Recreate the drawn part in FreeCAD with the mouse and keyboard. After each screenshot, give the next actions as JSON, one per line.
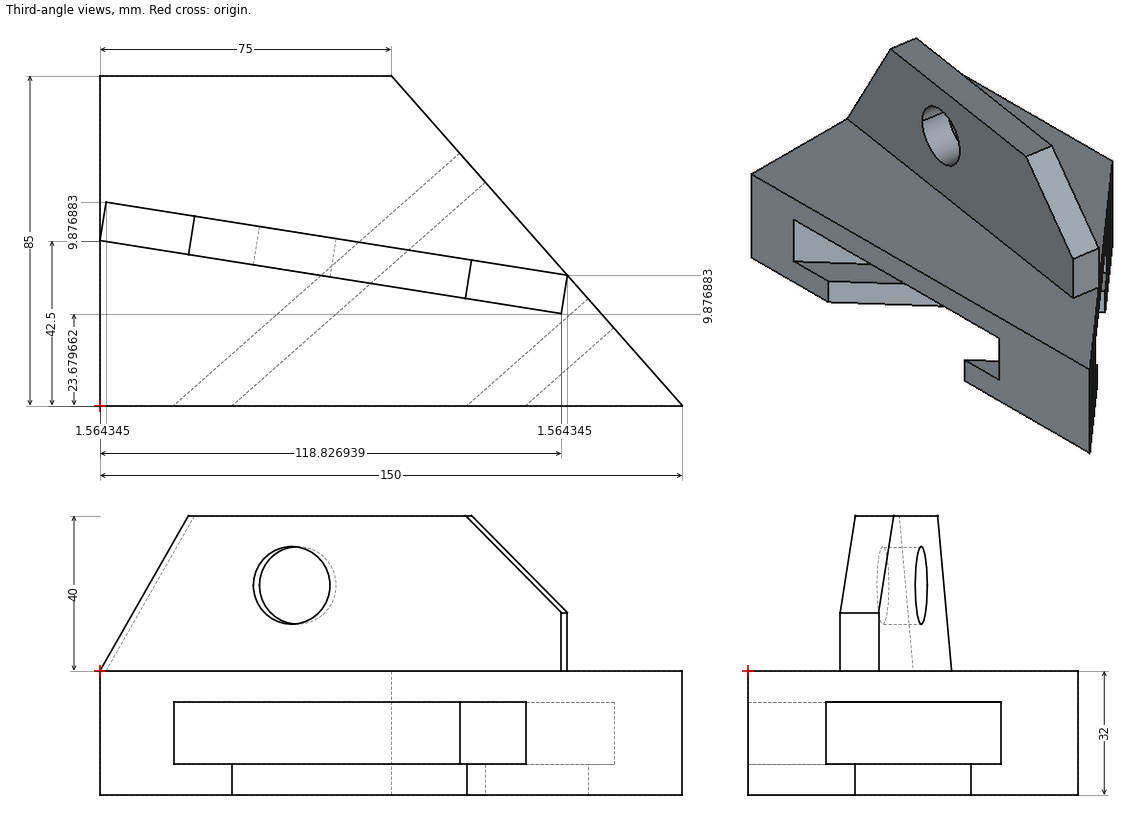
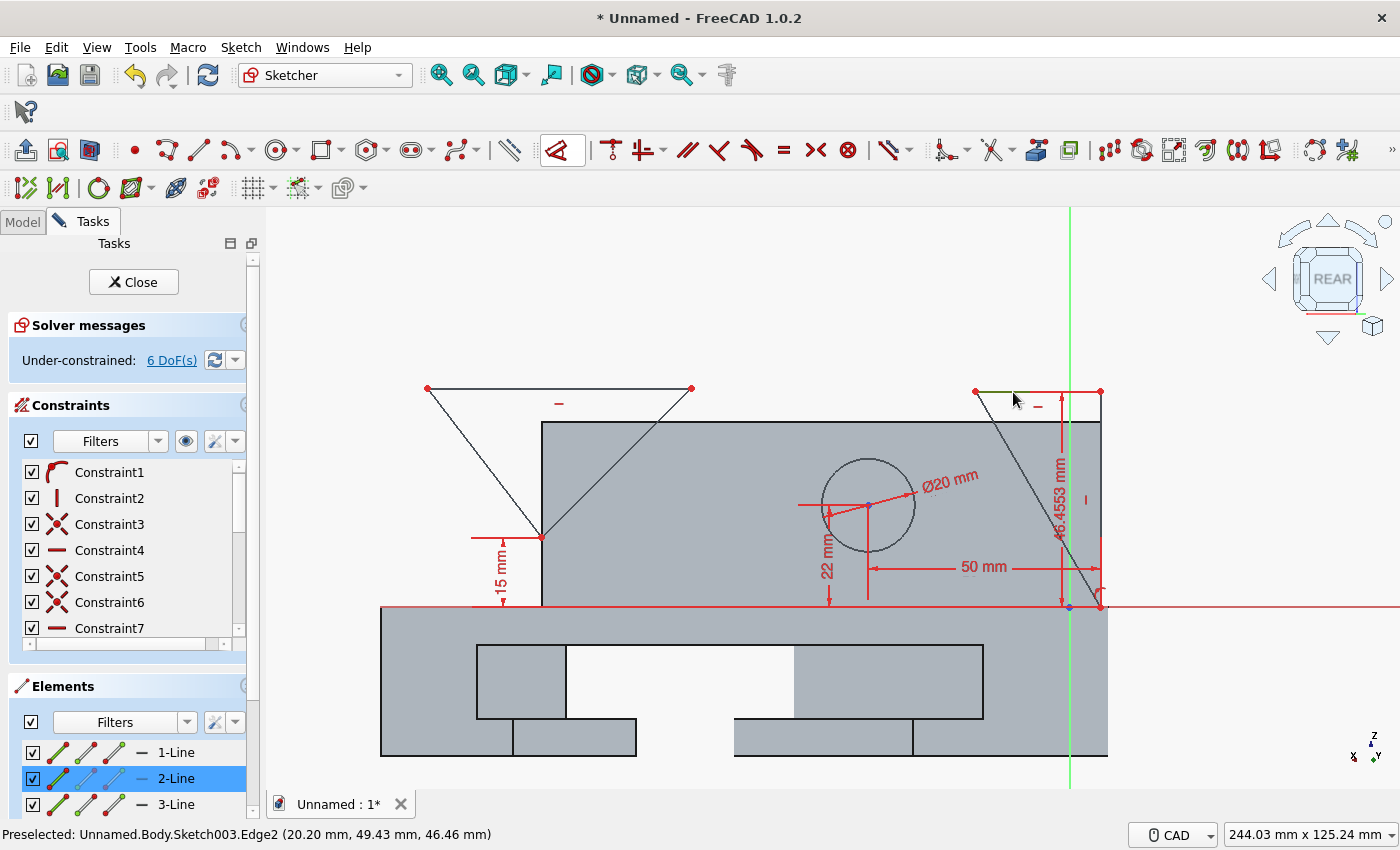
{"action": "key", "text": "l"}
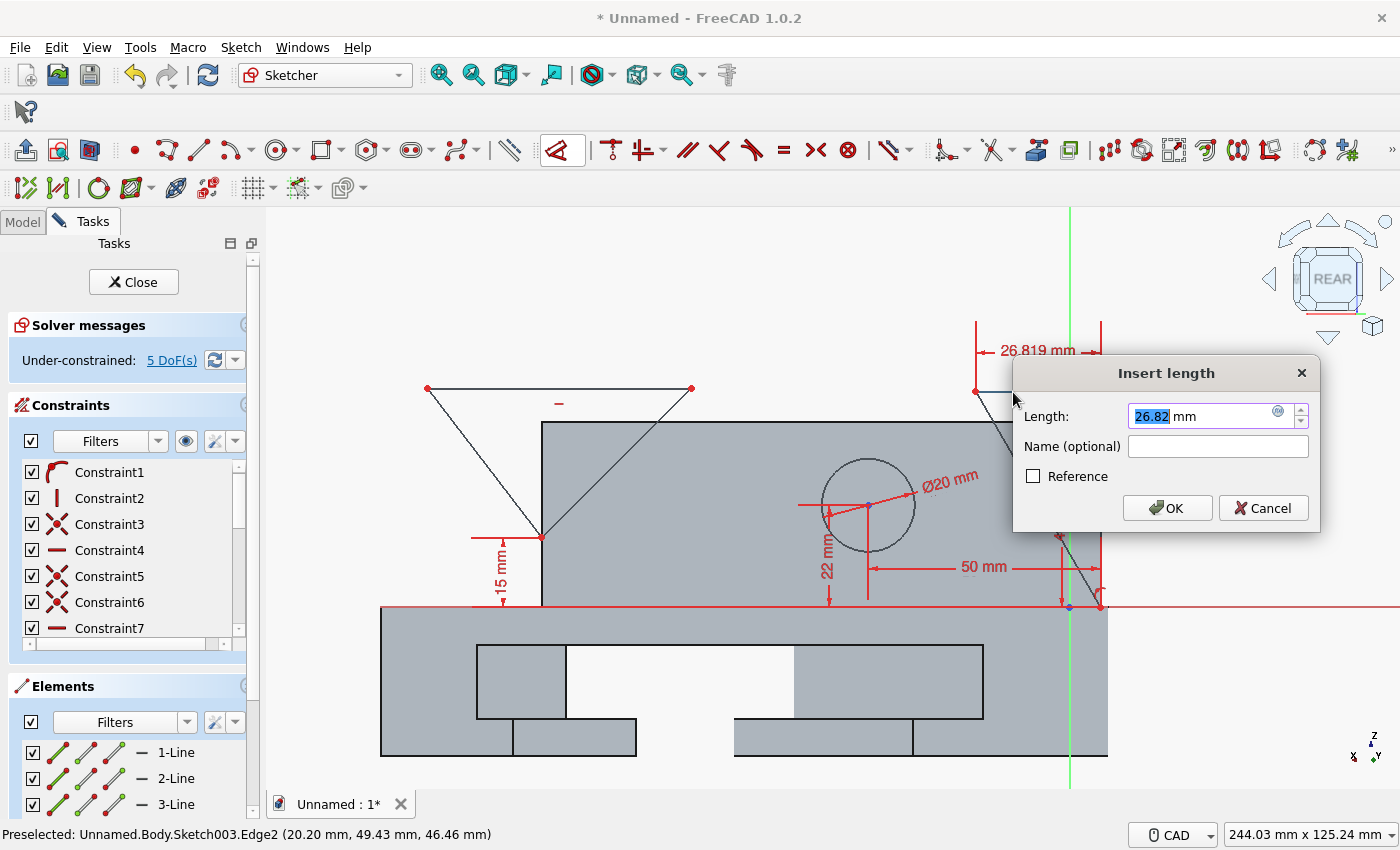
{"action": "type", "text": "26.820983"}
{"action": "key", "text": "Return"}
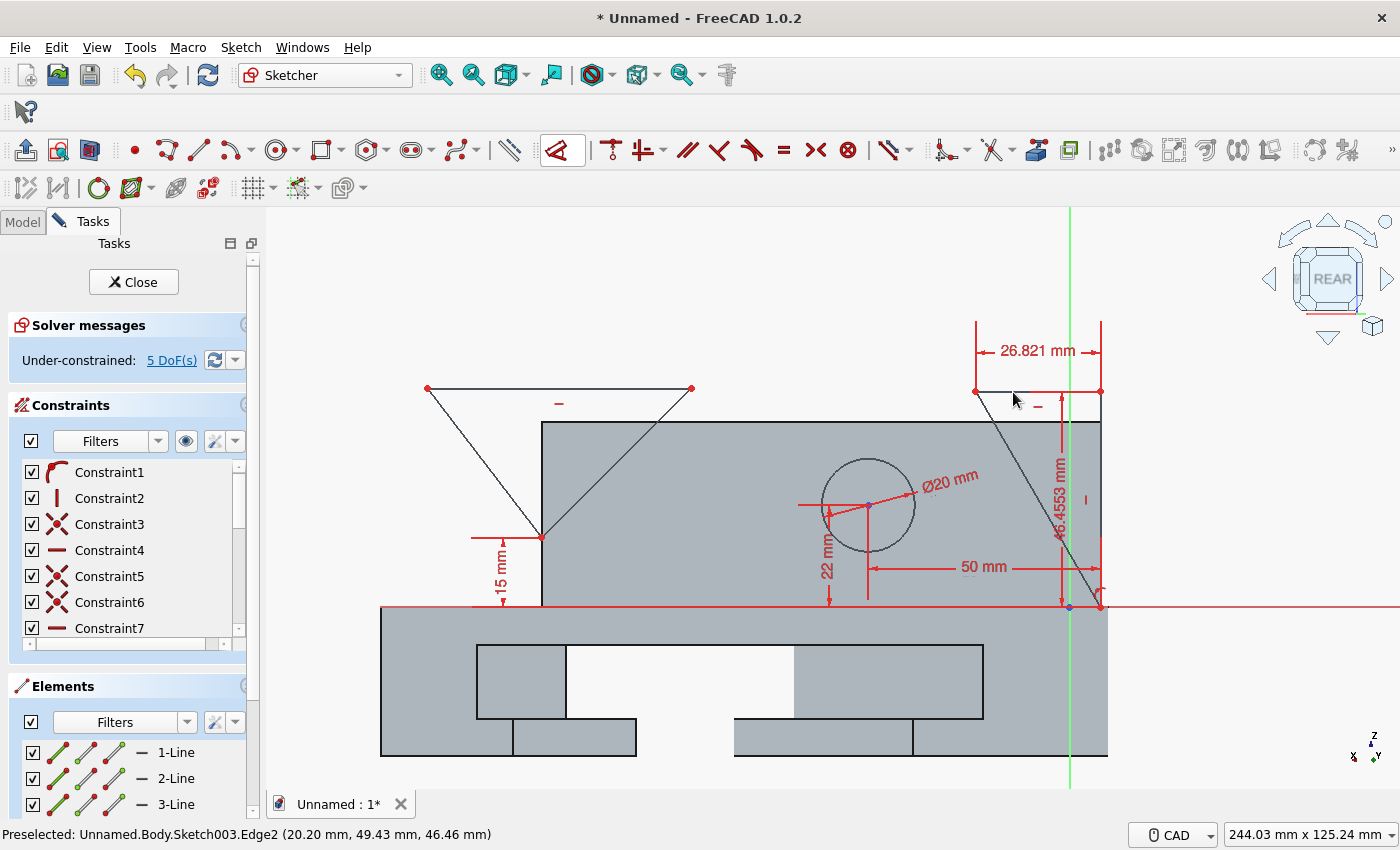
{"action": "left_click", "coordinate": [612, 389]}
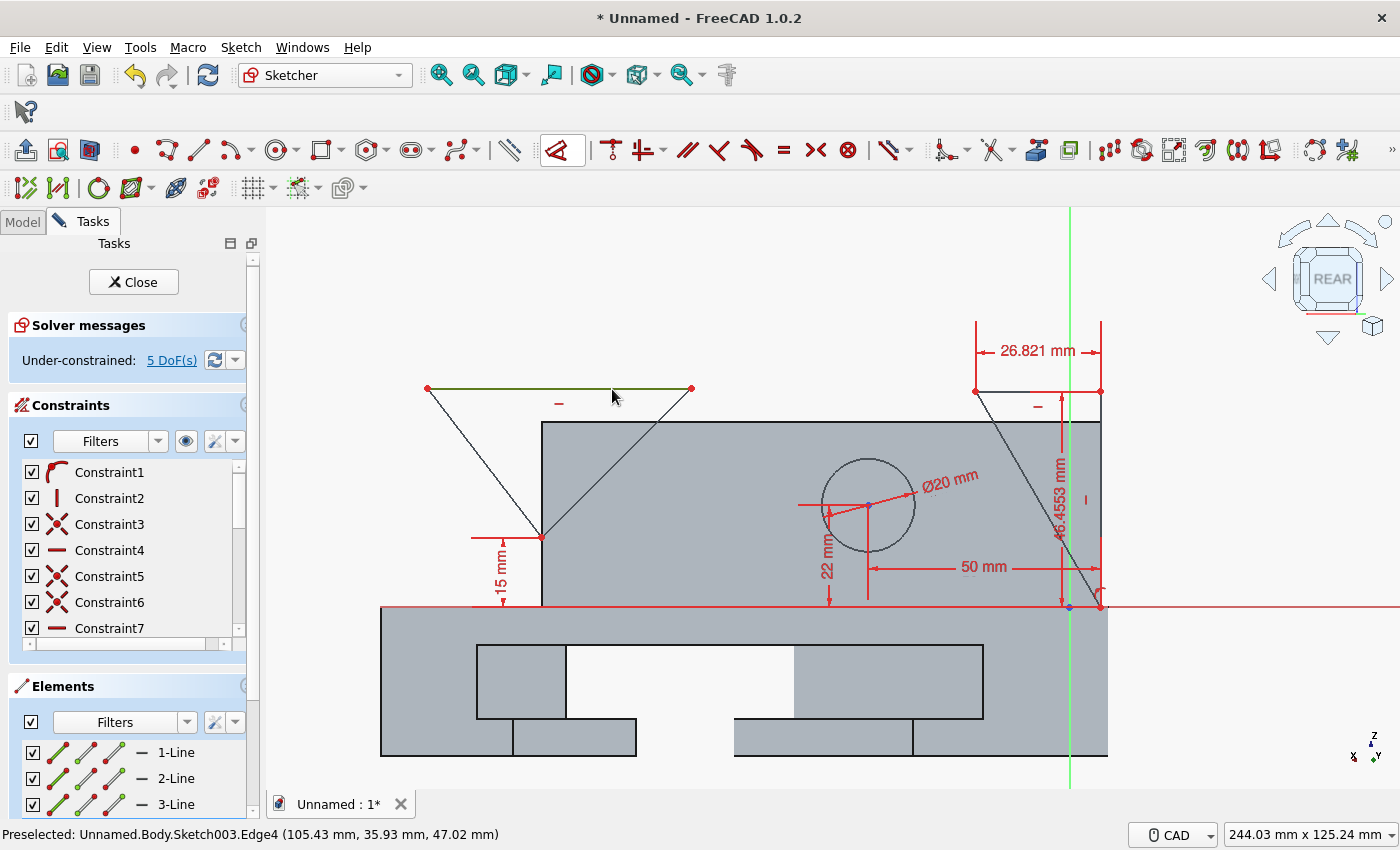
{"action": "key", "text": "l"}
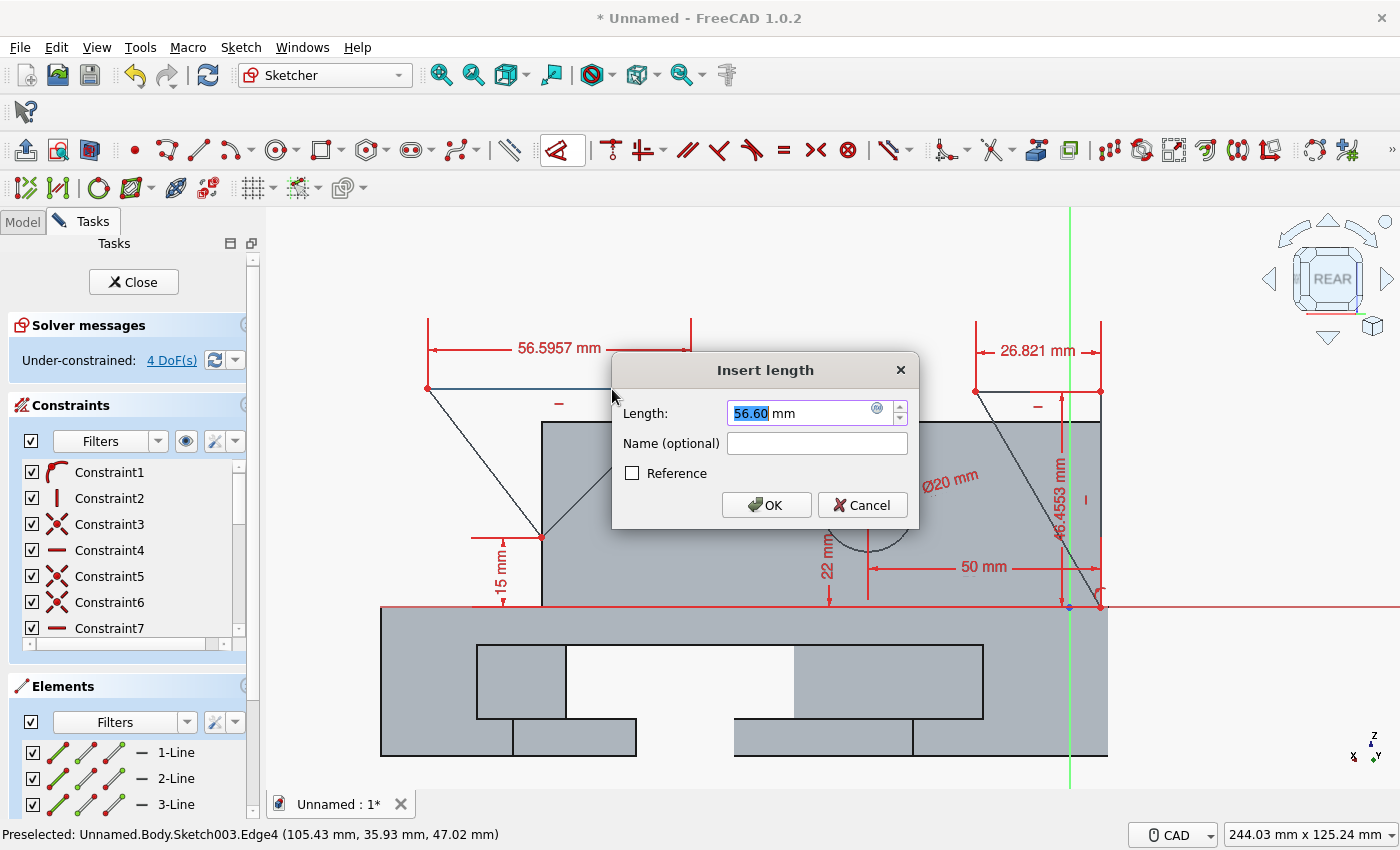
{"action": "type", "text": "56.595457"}
{"action": "key", "text": "Return"}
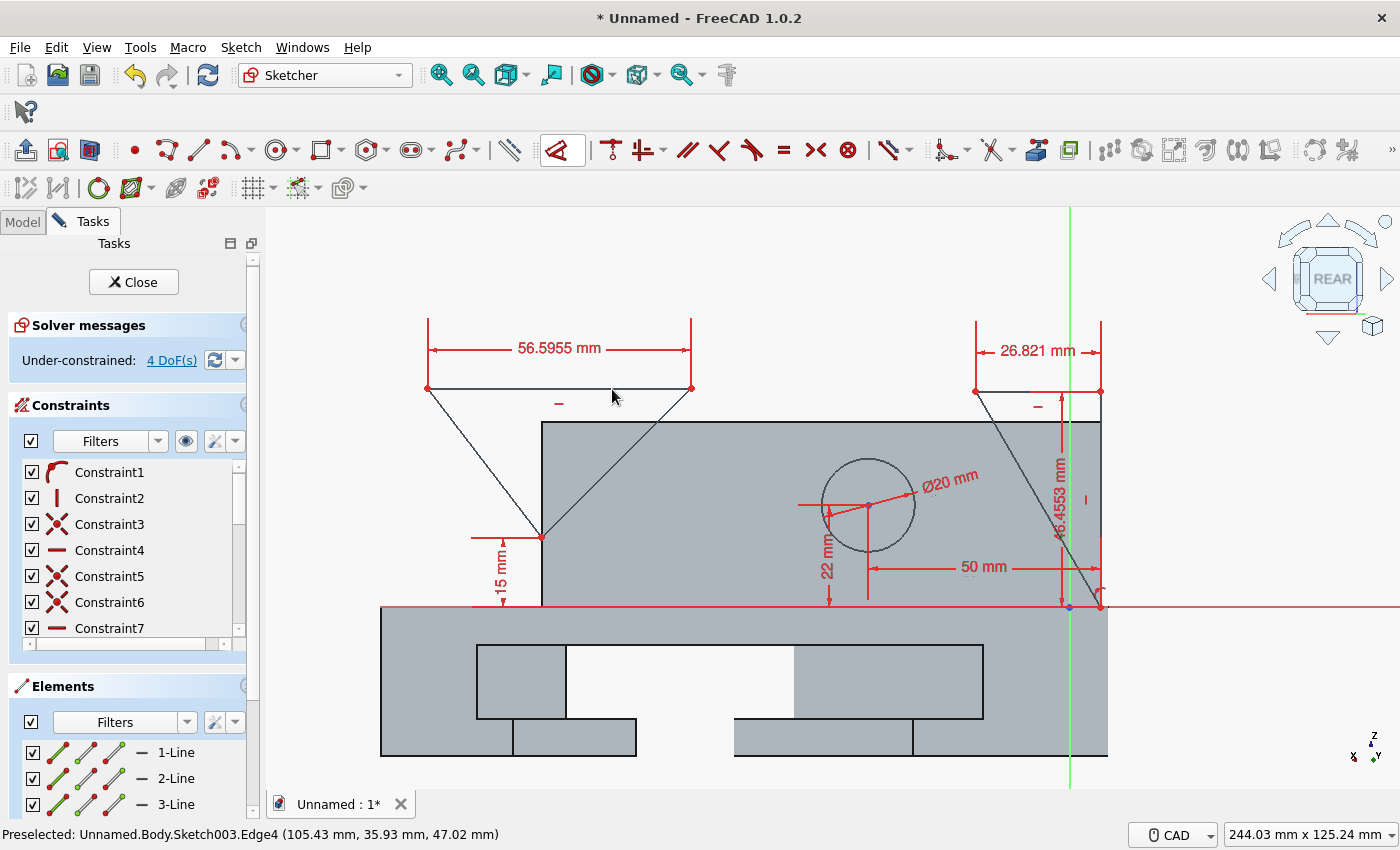
{"action": "scroll", "coordinate": [1101, 607], "scroll_direction": "up", "scroll_amount": 2}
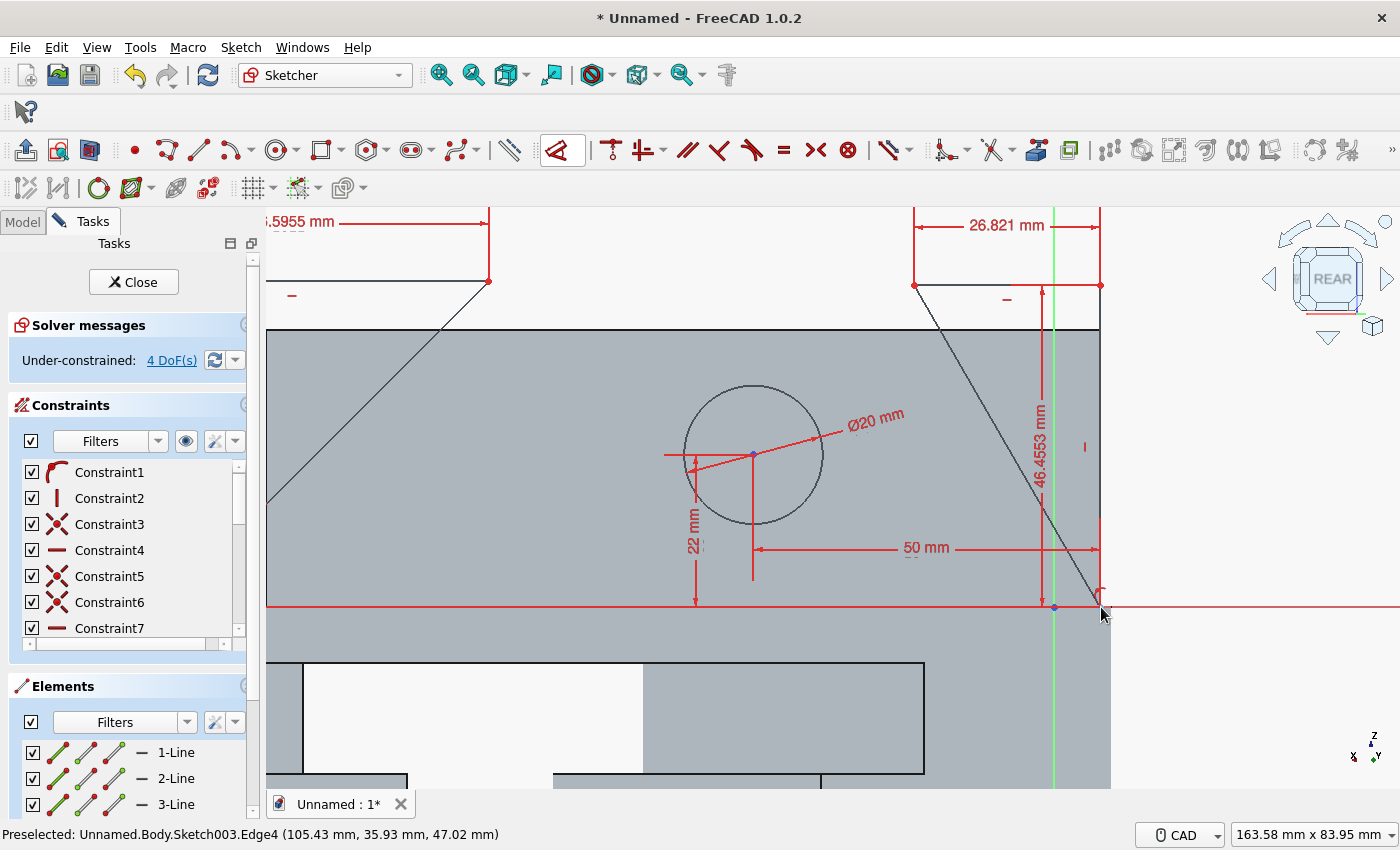
{"action": "left_click", "coordinate": [1100, 607]}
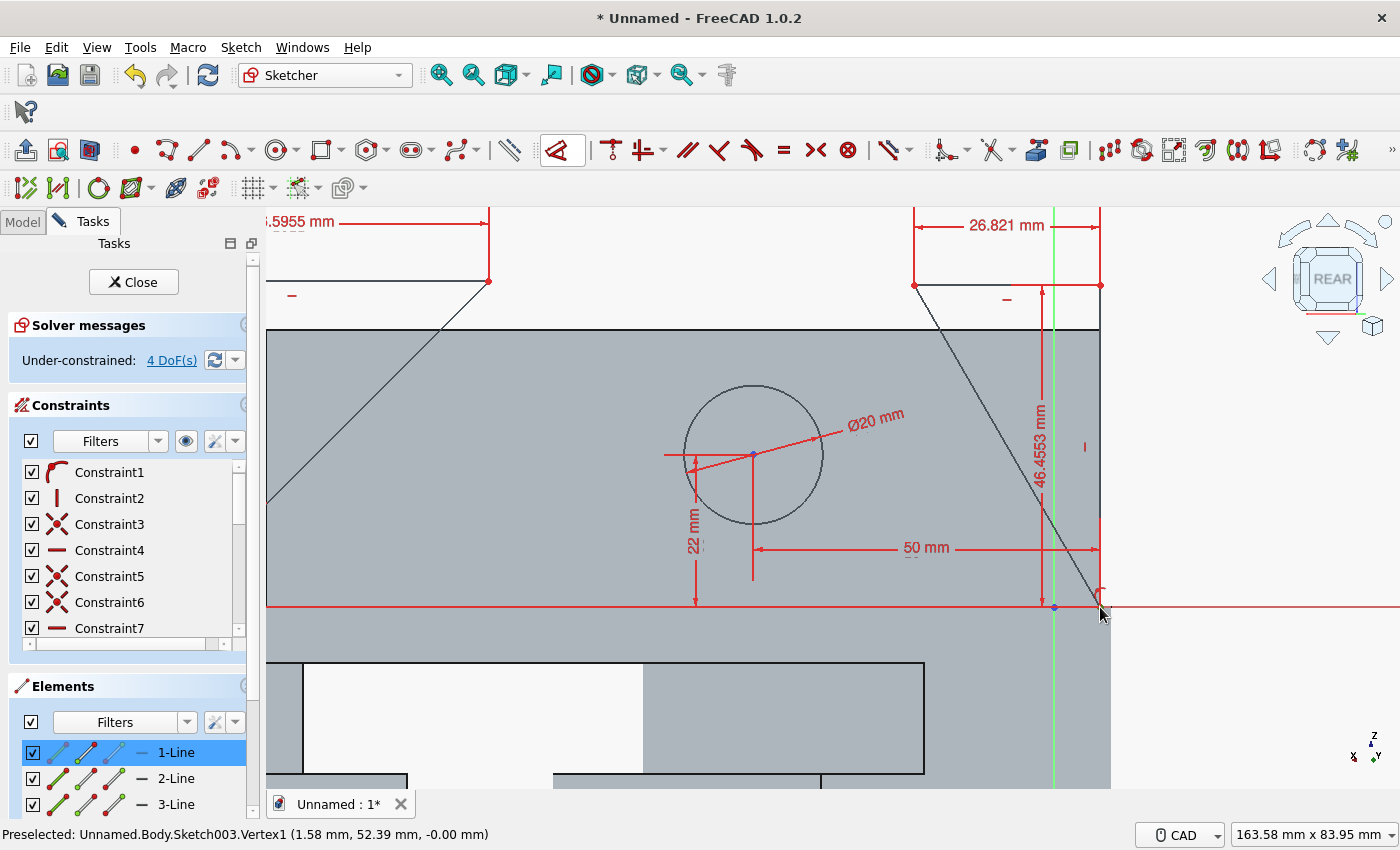
{"action": "key", "text": "l"}